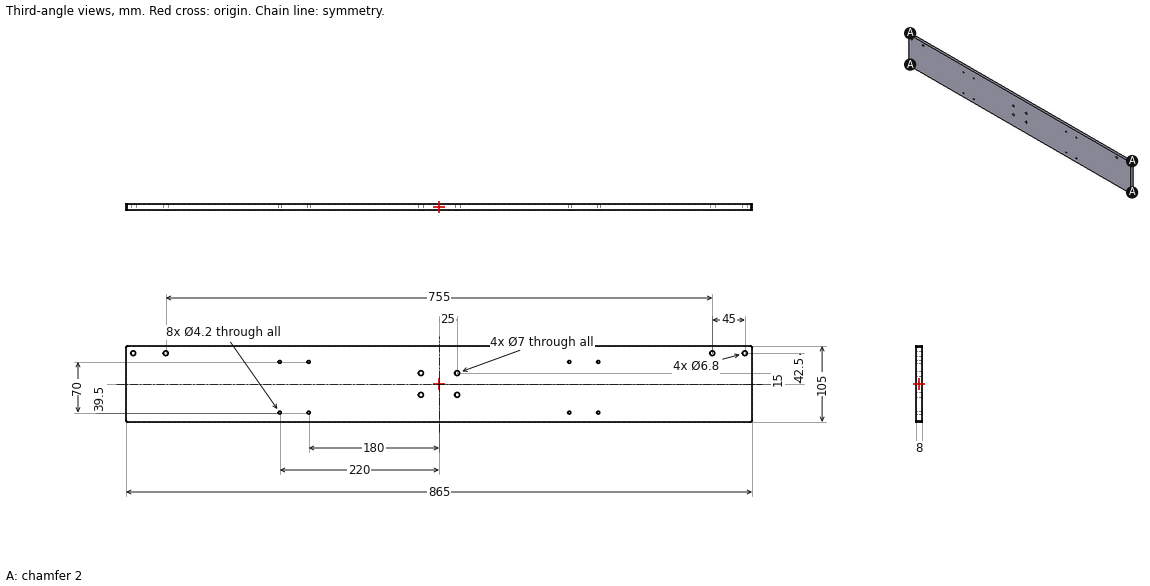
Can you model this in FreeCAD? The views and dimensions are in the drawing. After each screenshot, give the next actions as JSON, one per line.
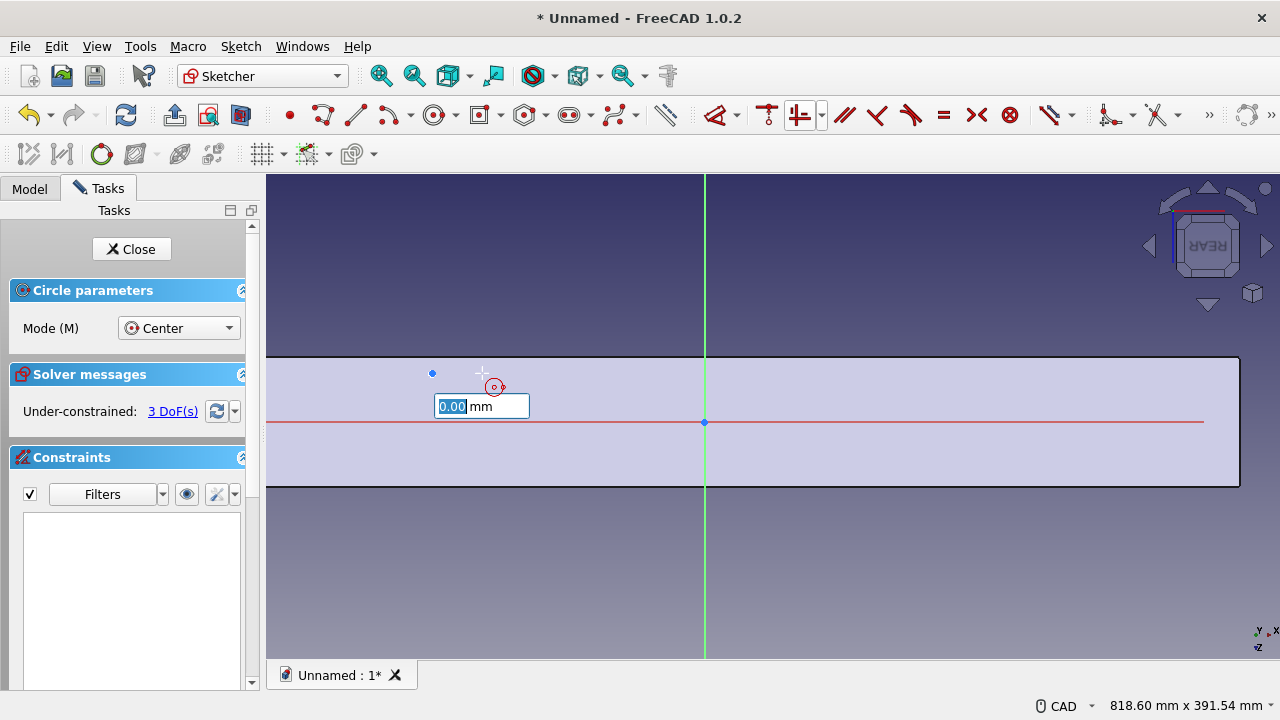
{"action": "scroll", "coordinate": [483, 372], "scroll_direction": "up", "scroll_amount": 10}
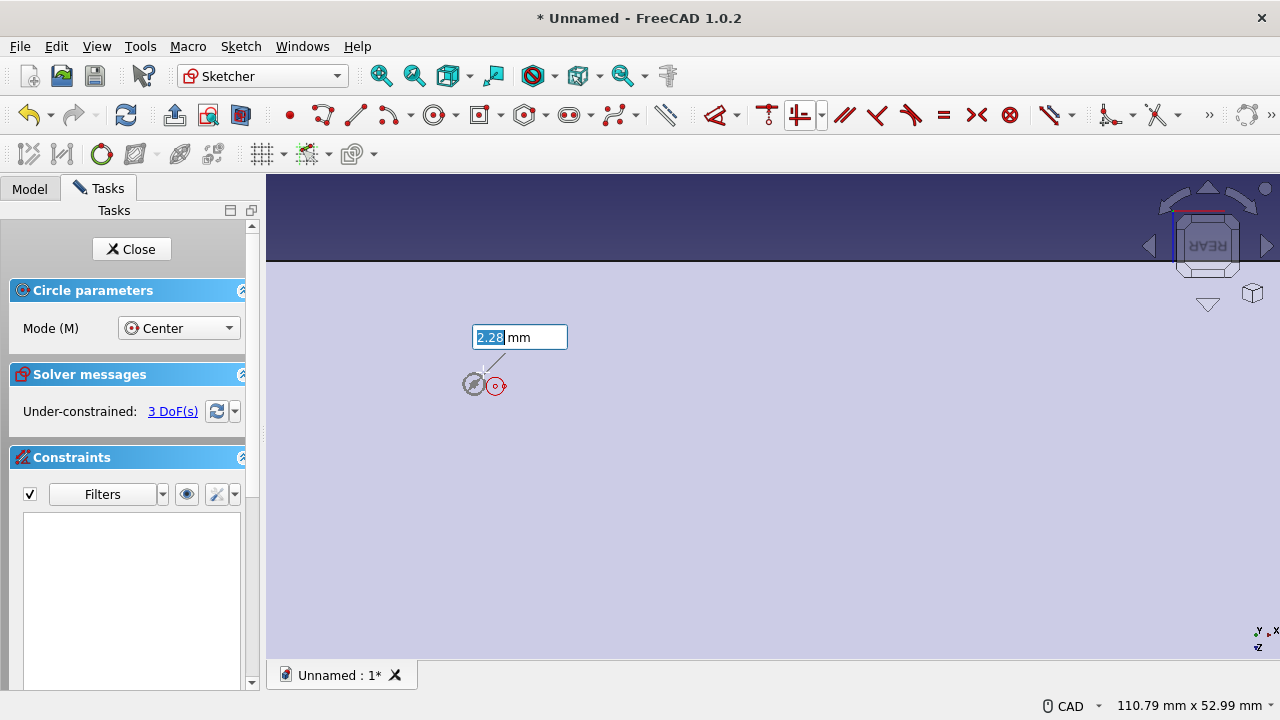
{"action": "left_click", "coordinate": [485, 366]}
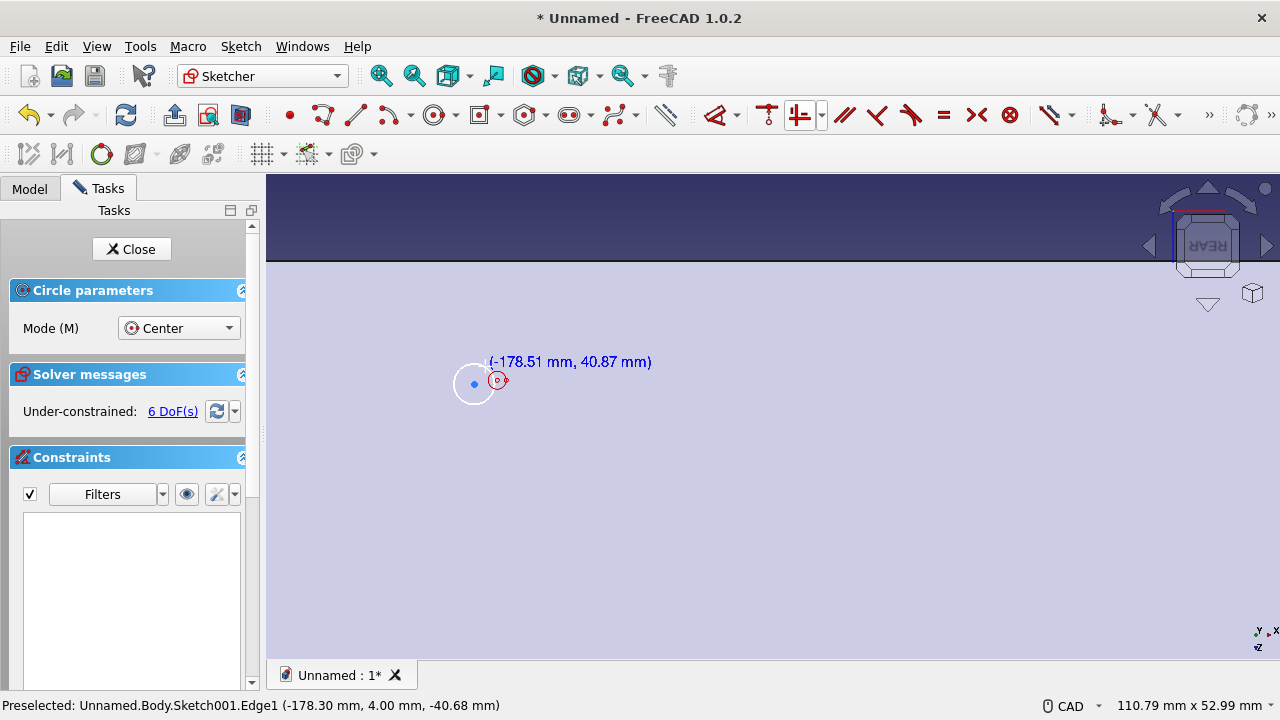
{"action": "scroll", "coordinate": [483, 372], "scroll_direction": "down", "scroll_amount": 10}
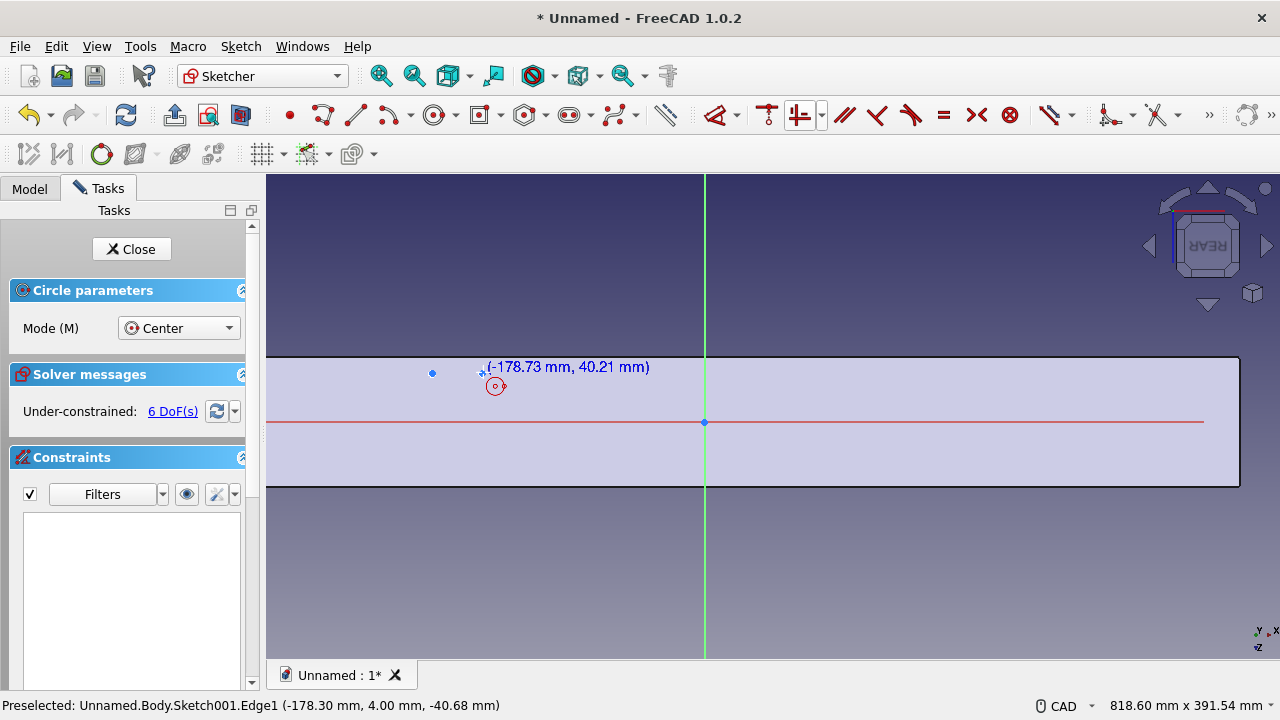
{"action": "scroll", "coordinate": [482, 460], "scroll_direction": "up", "scroll_amount": 11}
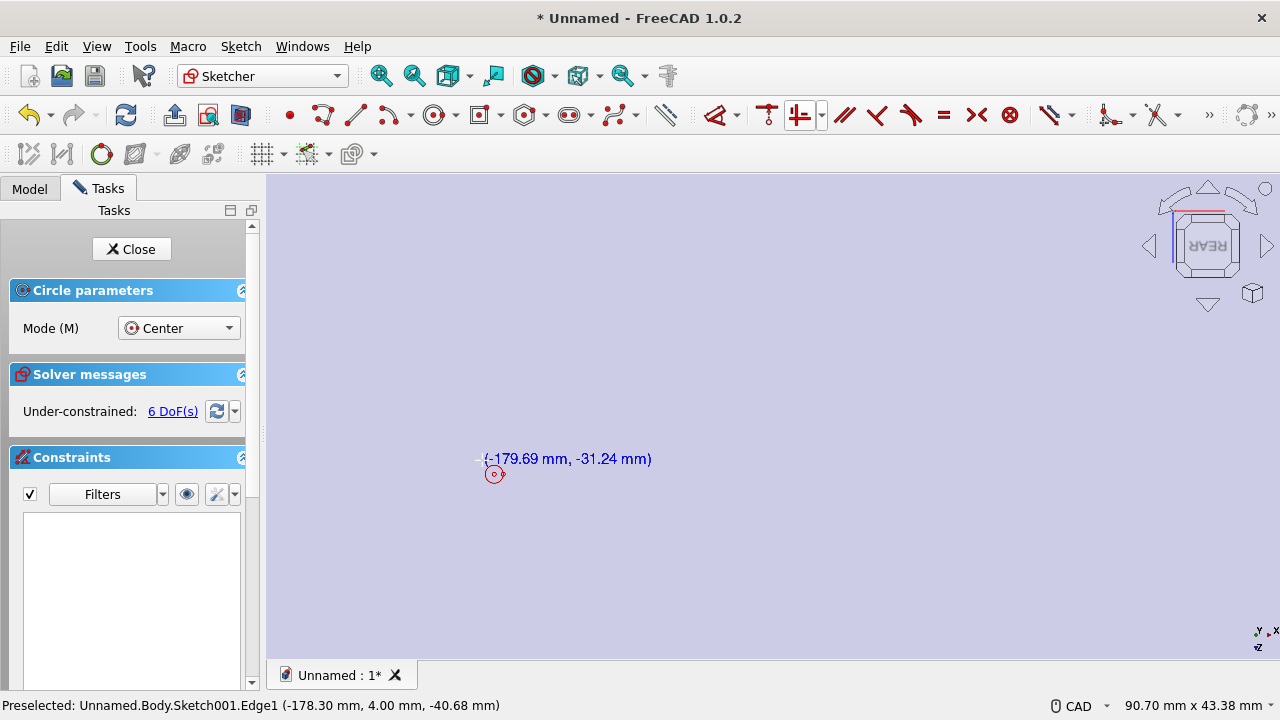
{"action": "scroll", "coordinate": [482, 460], "scroll_direction": "down", "scroll_amount": 11}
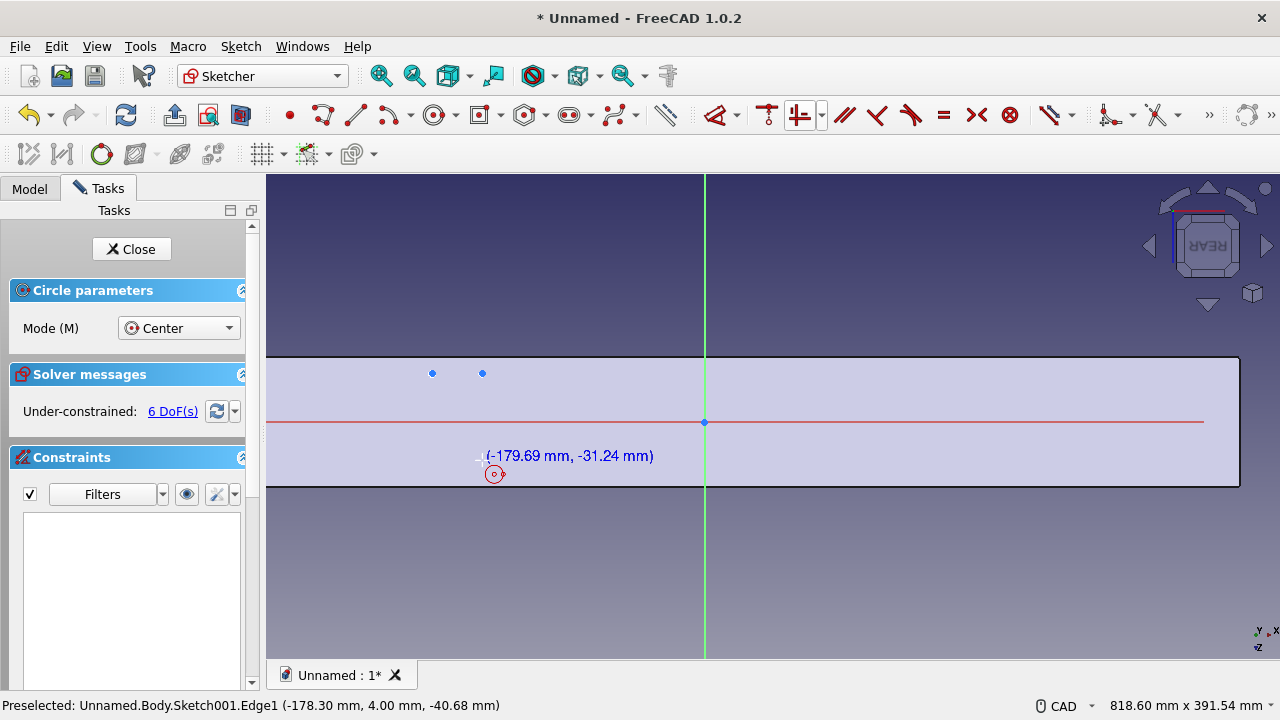
{"action": "left_click", "coordinate": [482, 460]}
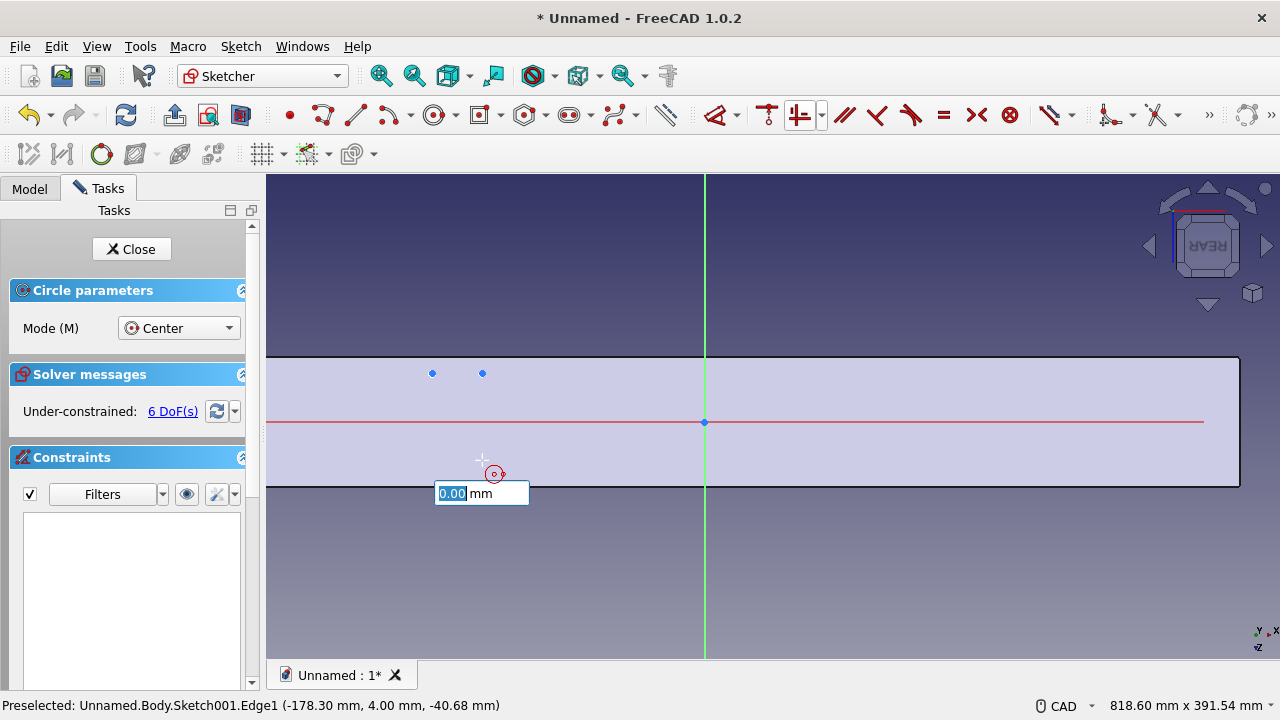
{"action": "scroll", "coordinate": [483, 458], "scroll_direction": "up", "scroll_amount": 10}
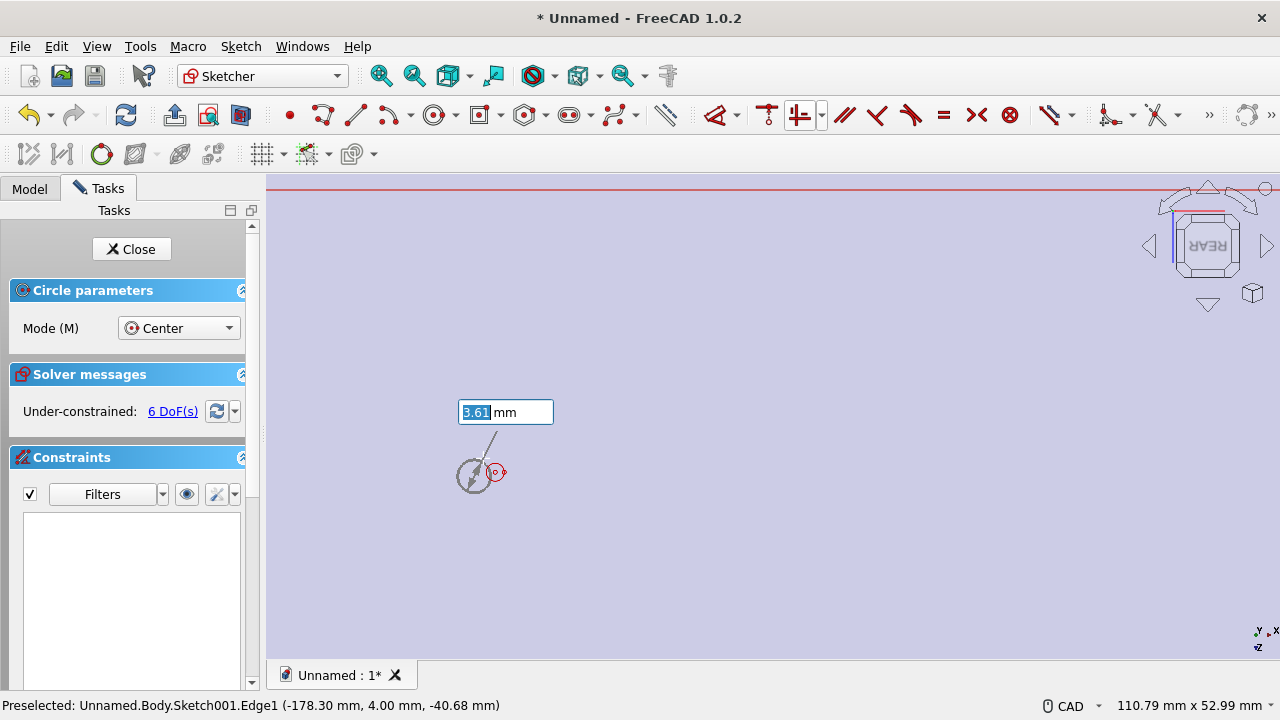
{"action": "left_click", "coordinate": [485, 456]}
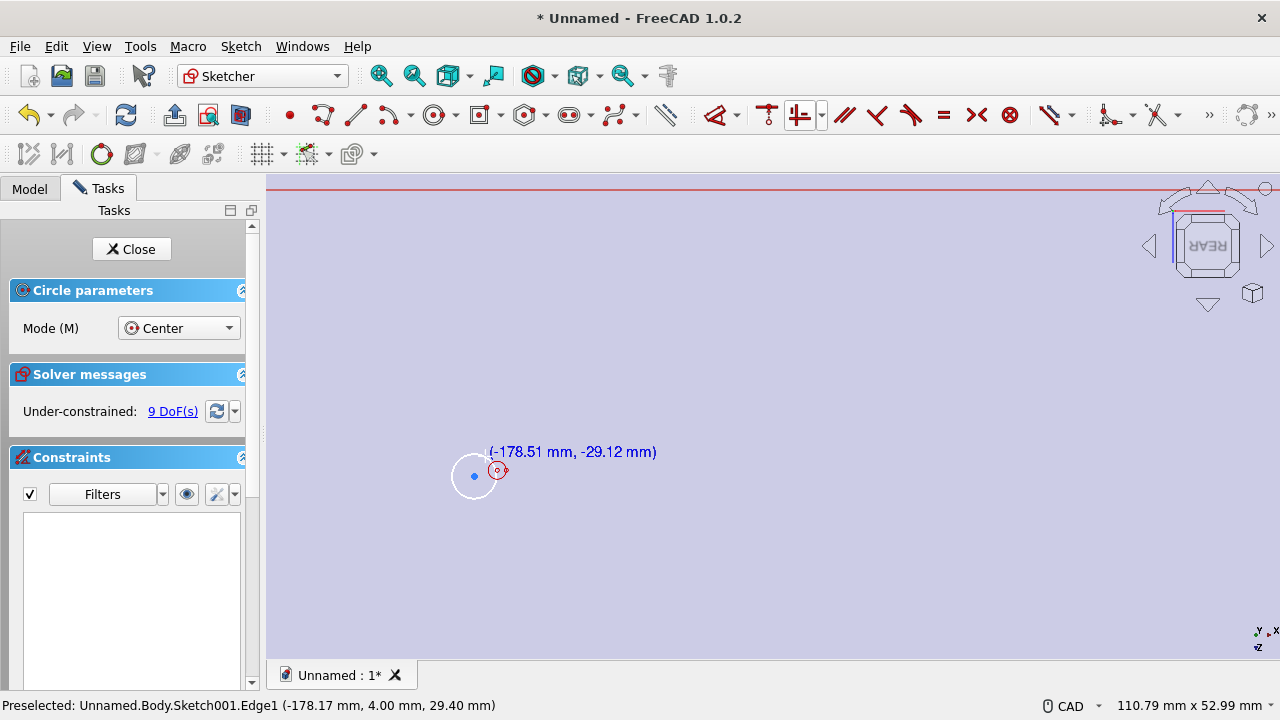
{"action": "scroll", "coordinate": [483, 458], "scroll_direction": "down", "scroll_amount": 10}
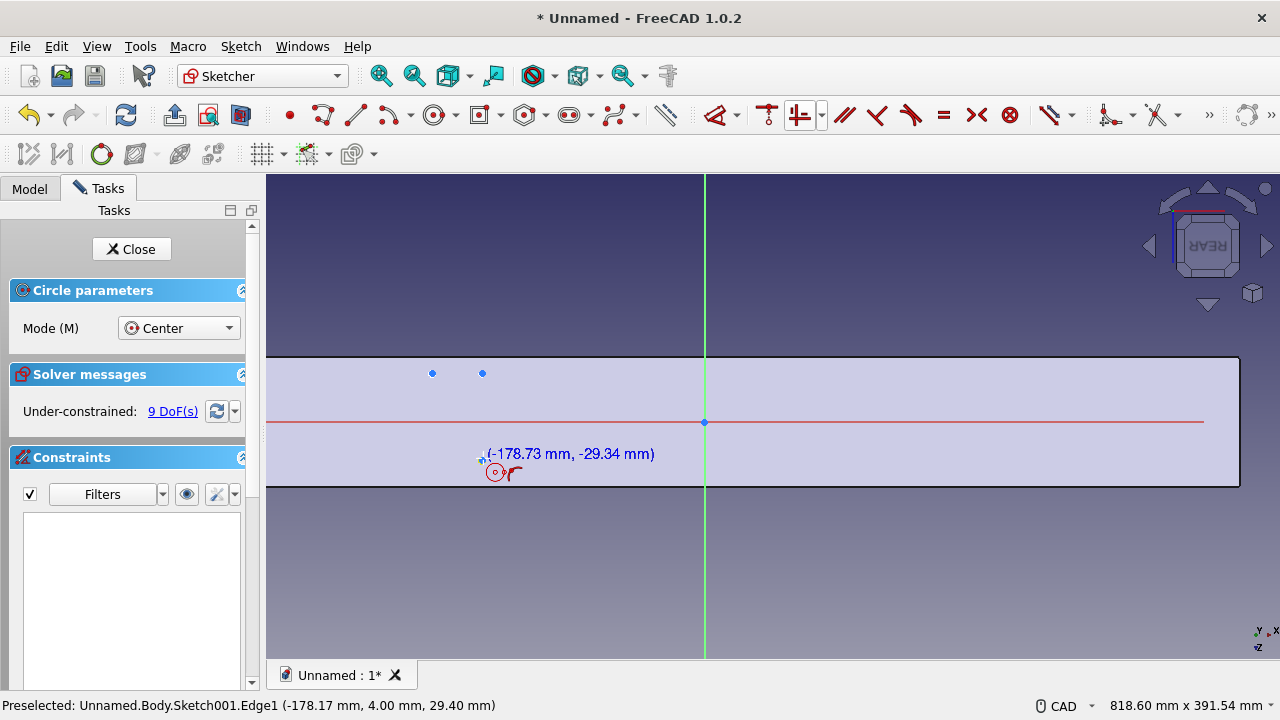
{"action": "scroll", "coordinate": [432, 460], "scroll_direction": "up", "scroll_amount": 11}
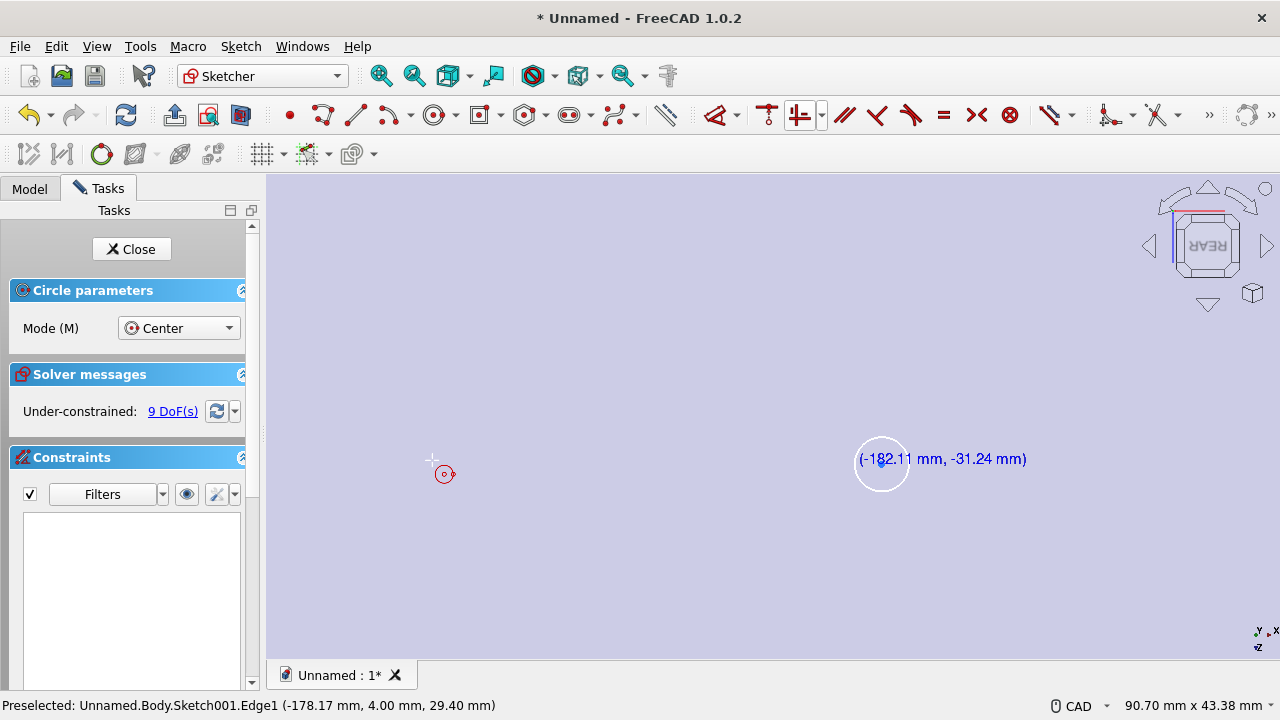
{"action": "scroll", "coordinate": [432, 460], "scroll_direction": "down", "scroll_amount": 11}